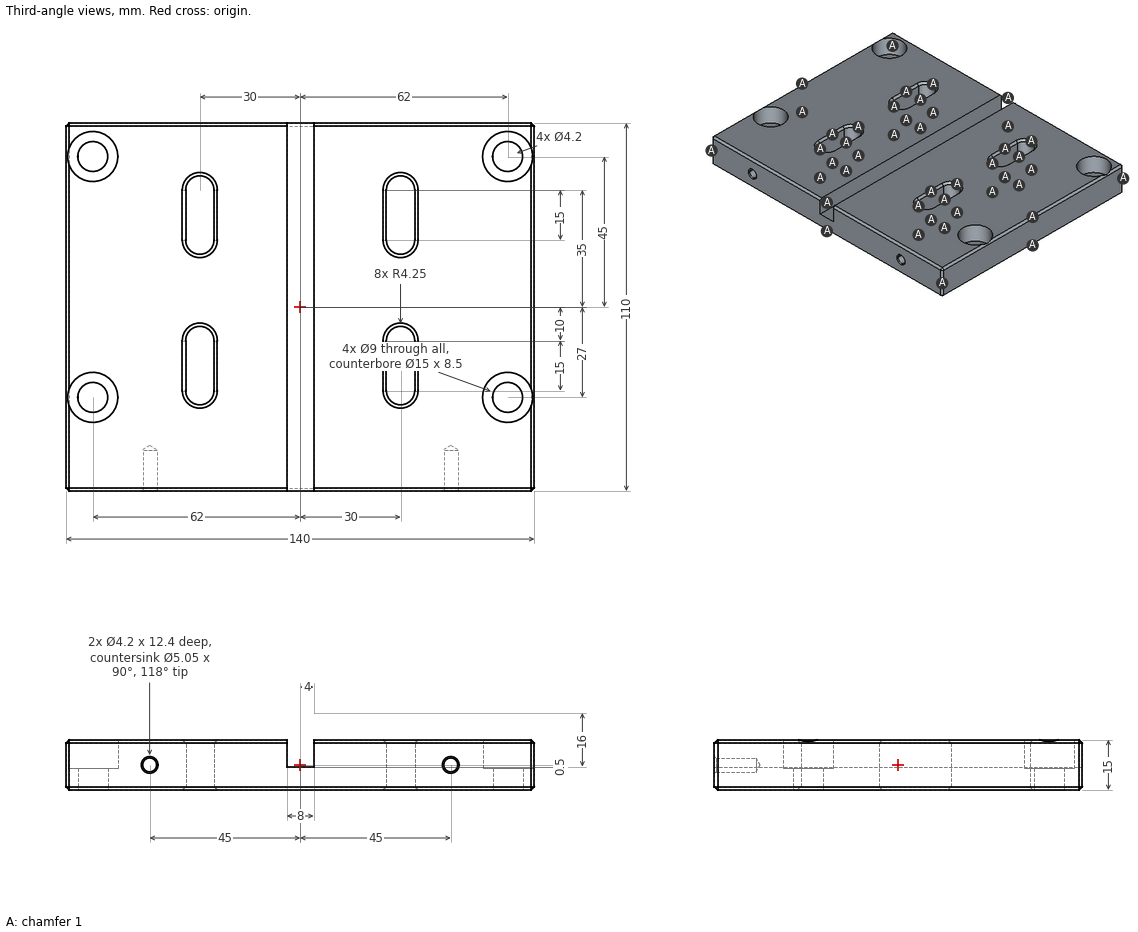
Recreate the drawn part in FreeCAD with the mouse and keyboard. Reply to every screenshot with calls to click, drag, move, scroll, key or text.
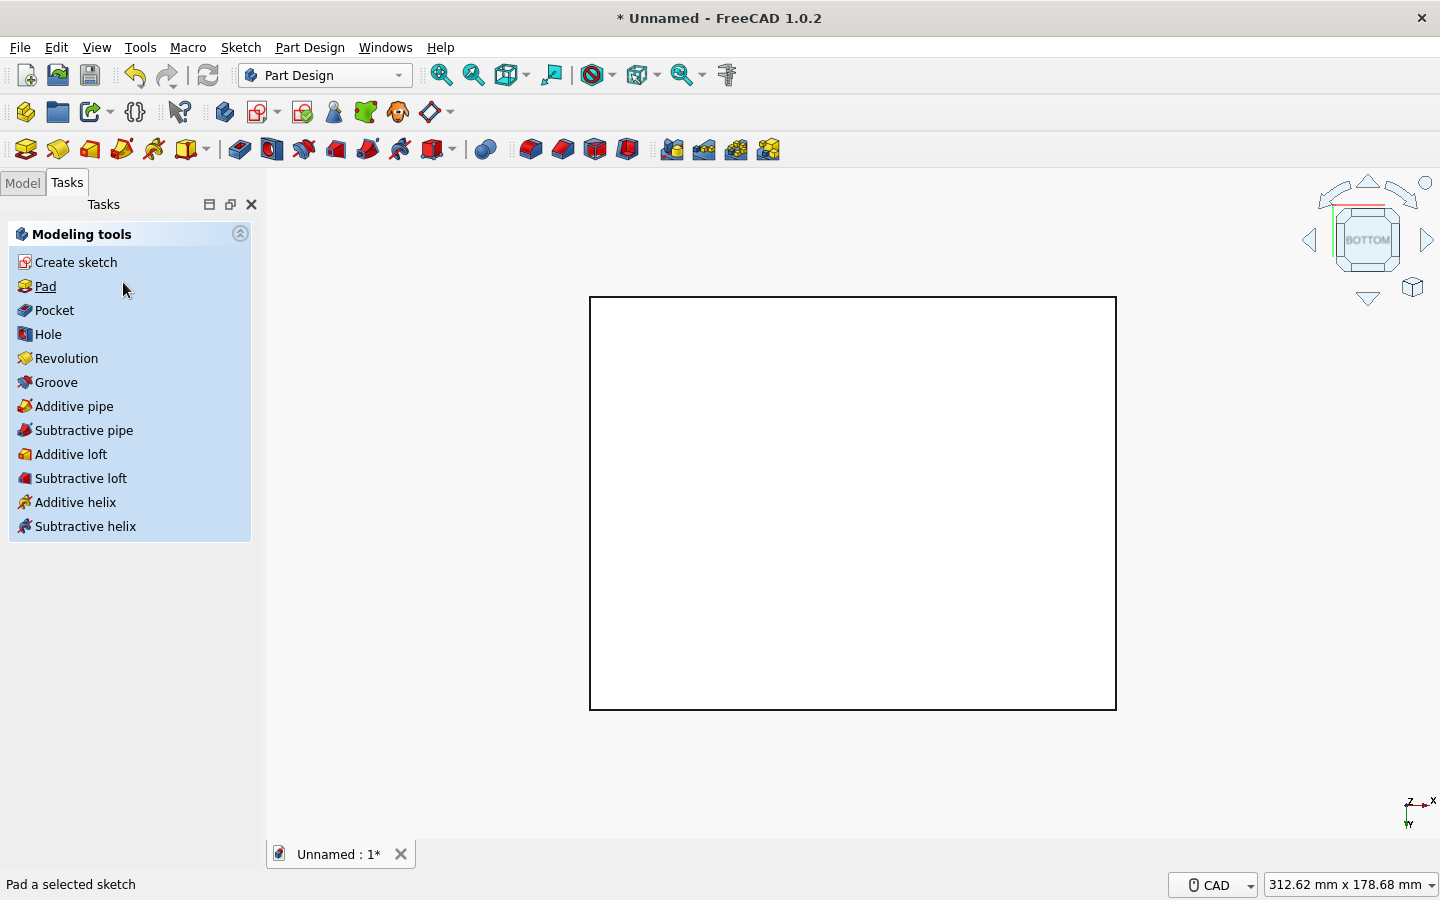
click(240, 150)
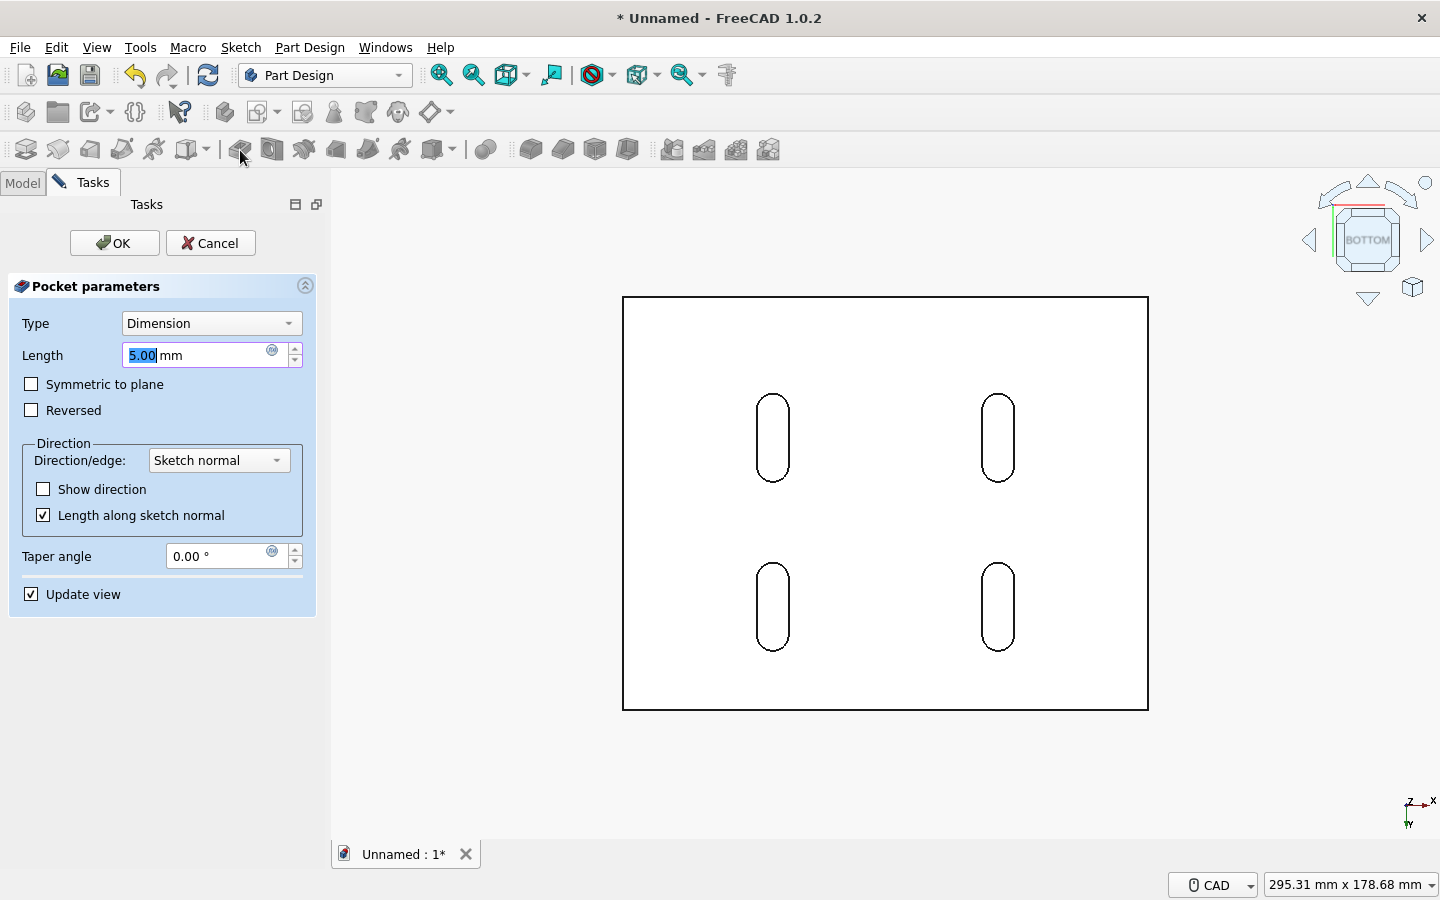
click(212, 324)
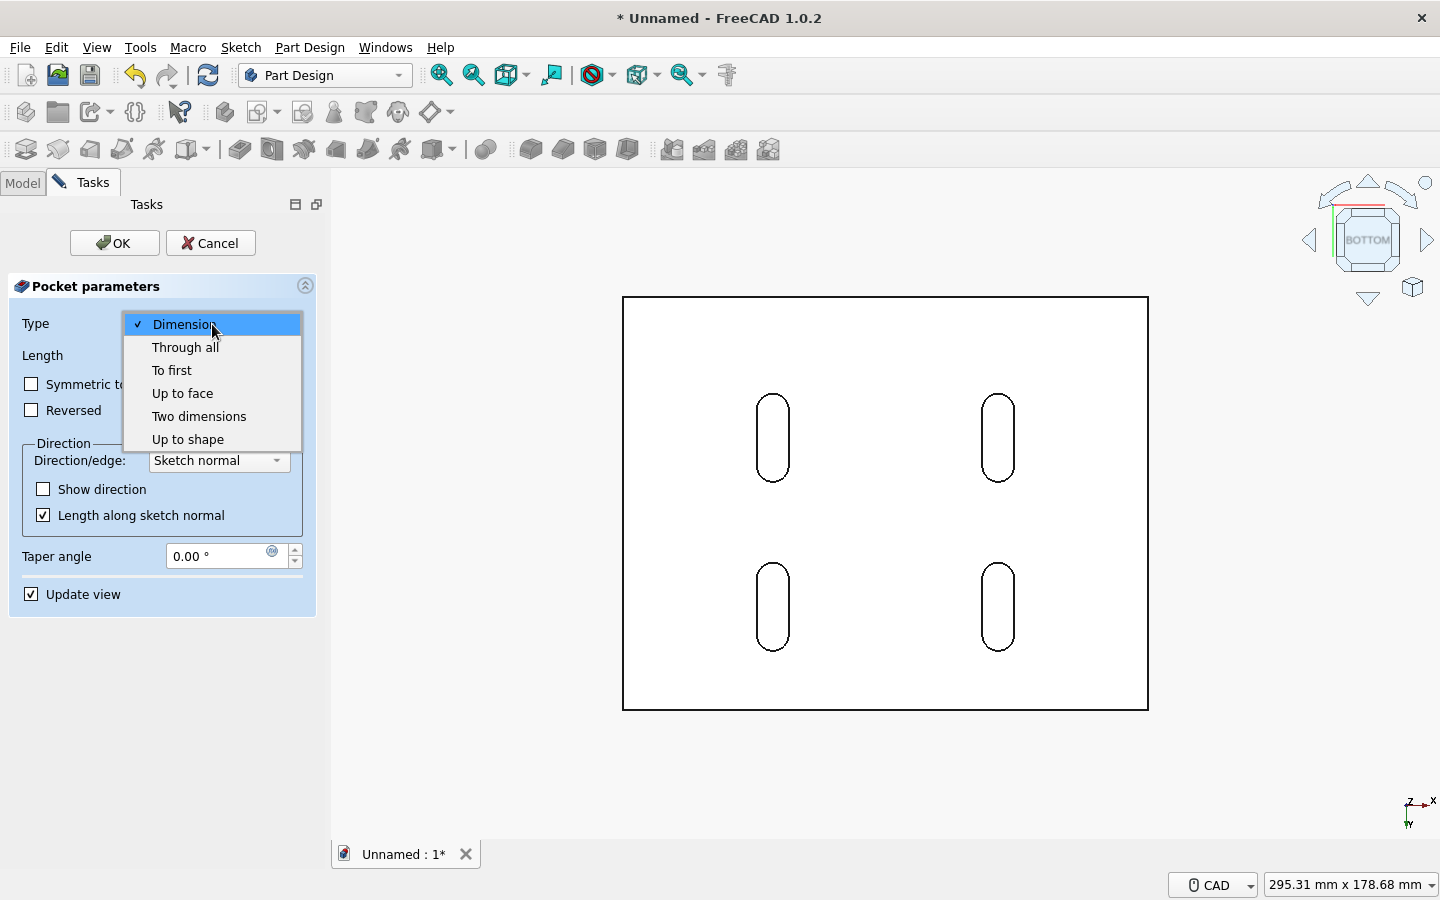
click(212, 348)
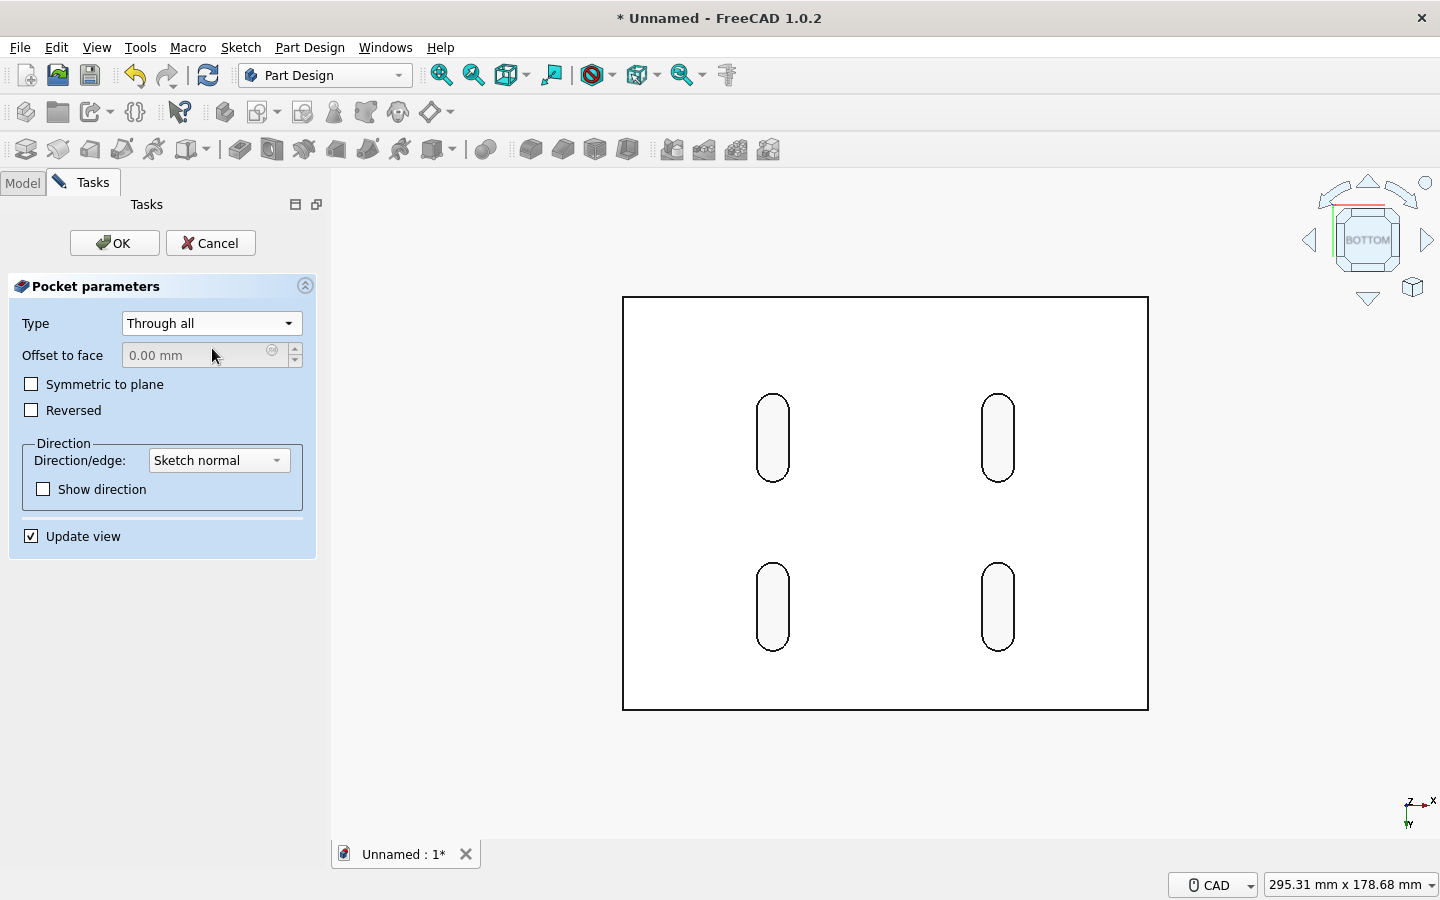
click(115, 243)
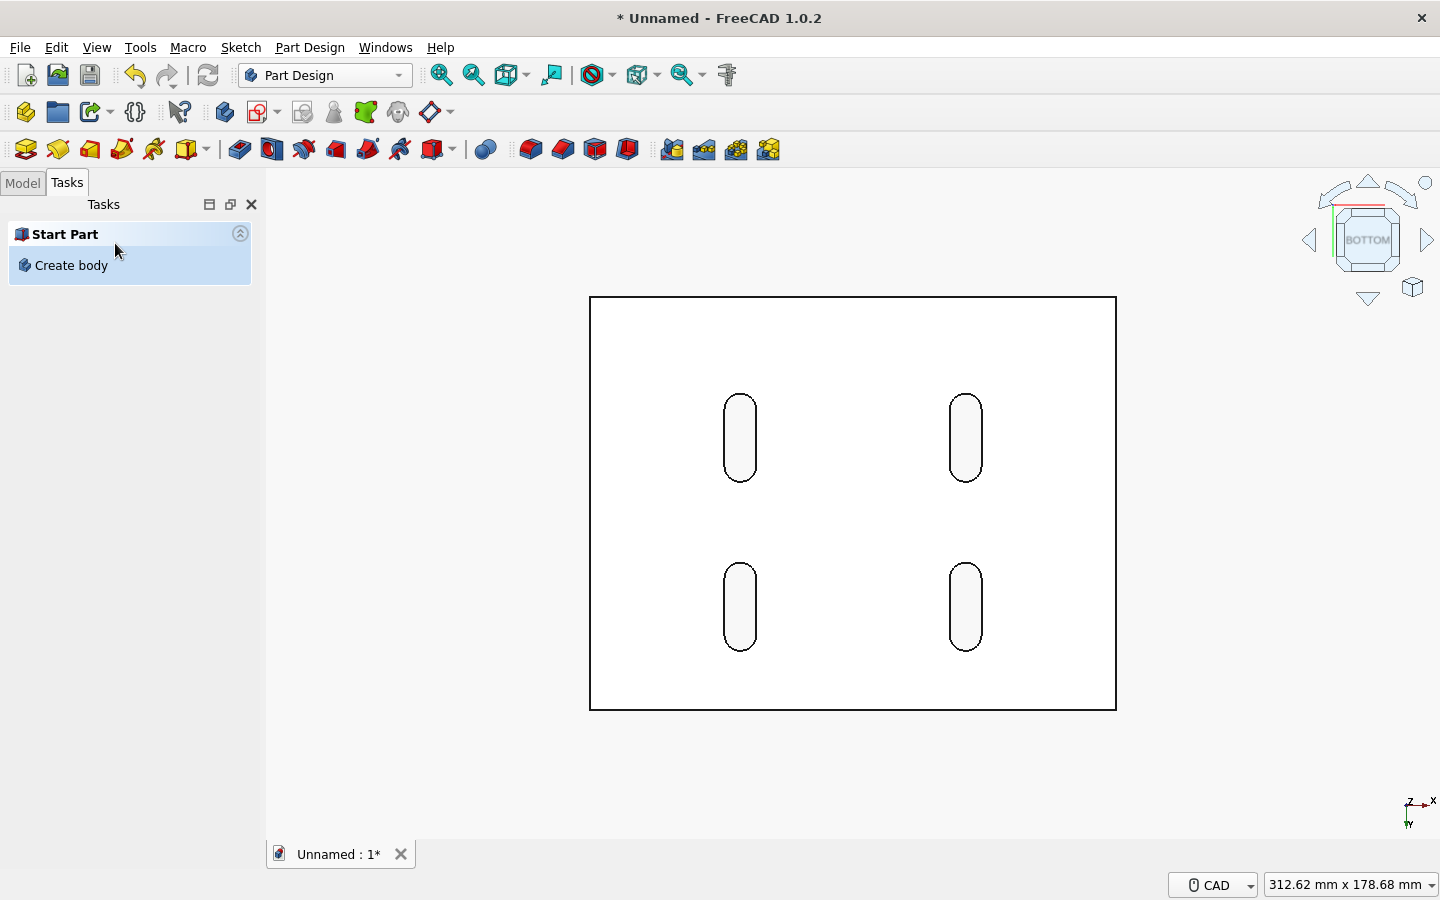
click(853, 503)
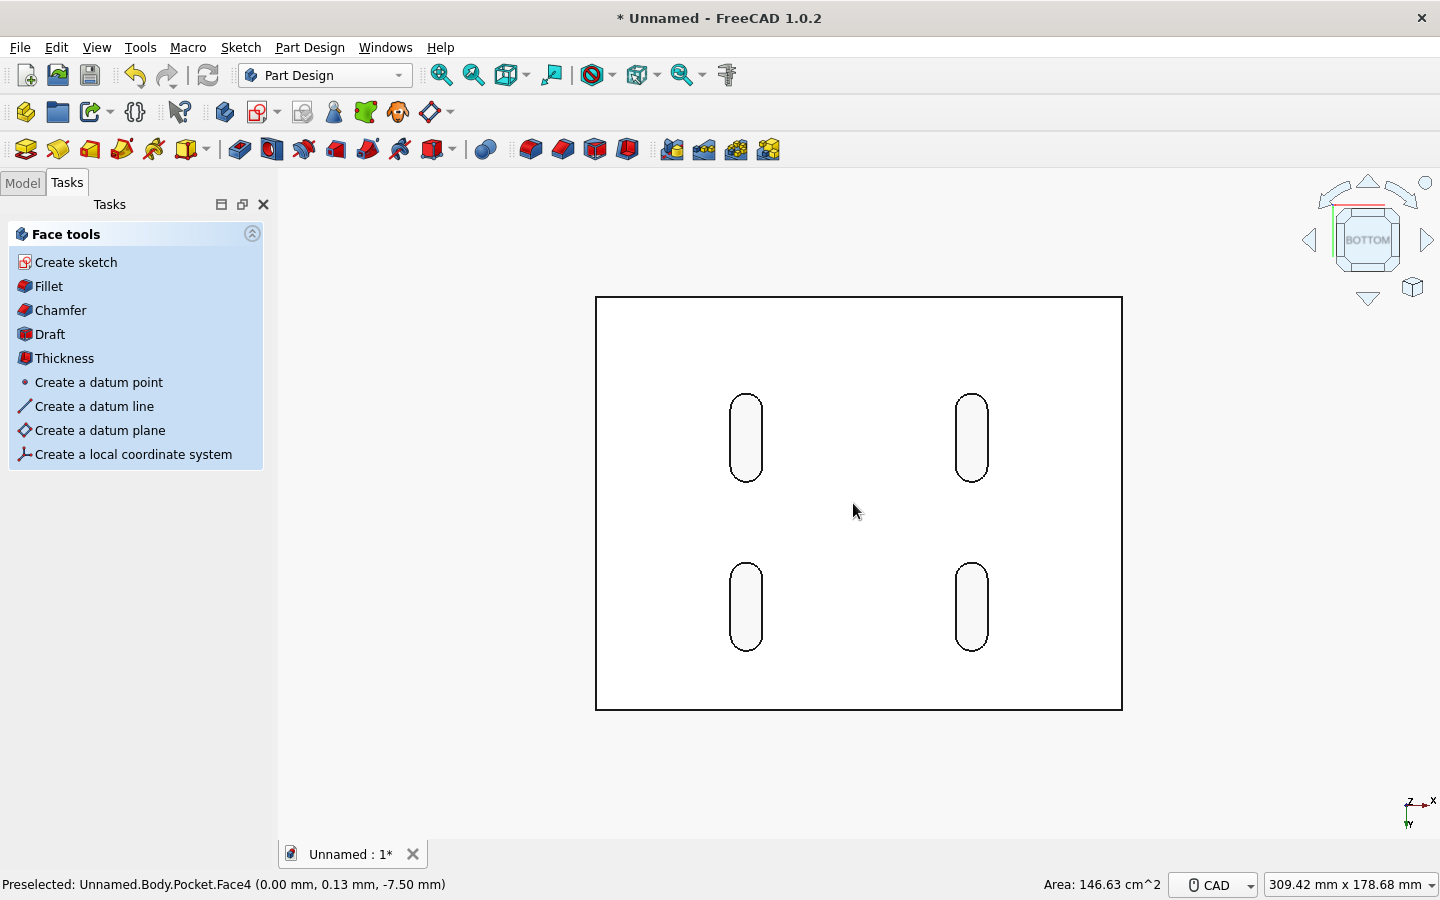
key(0)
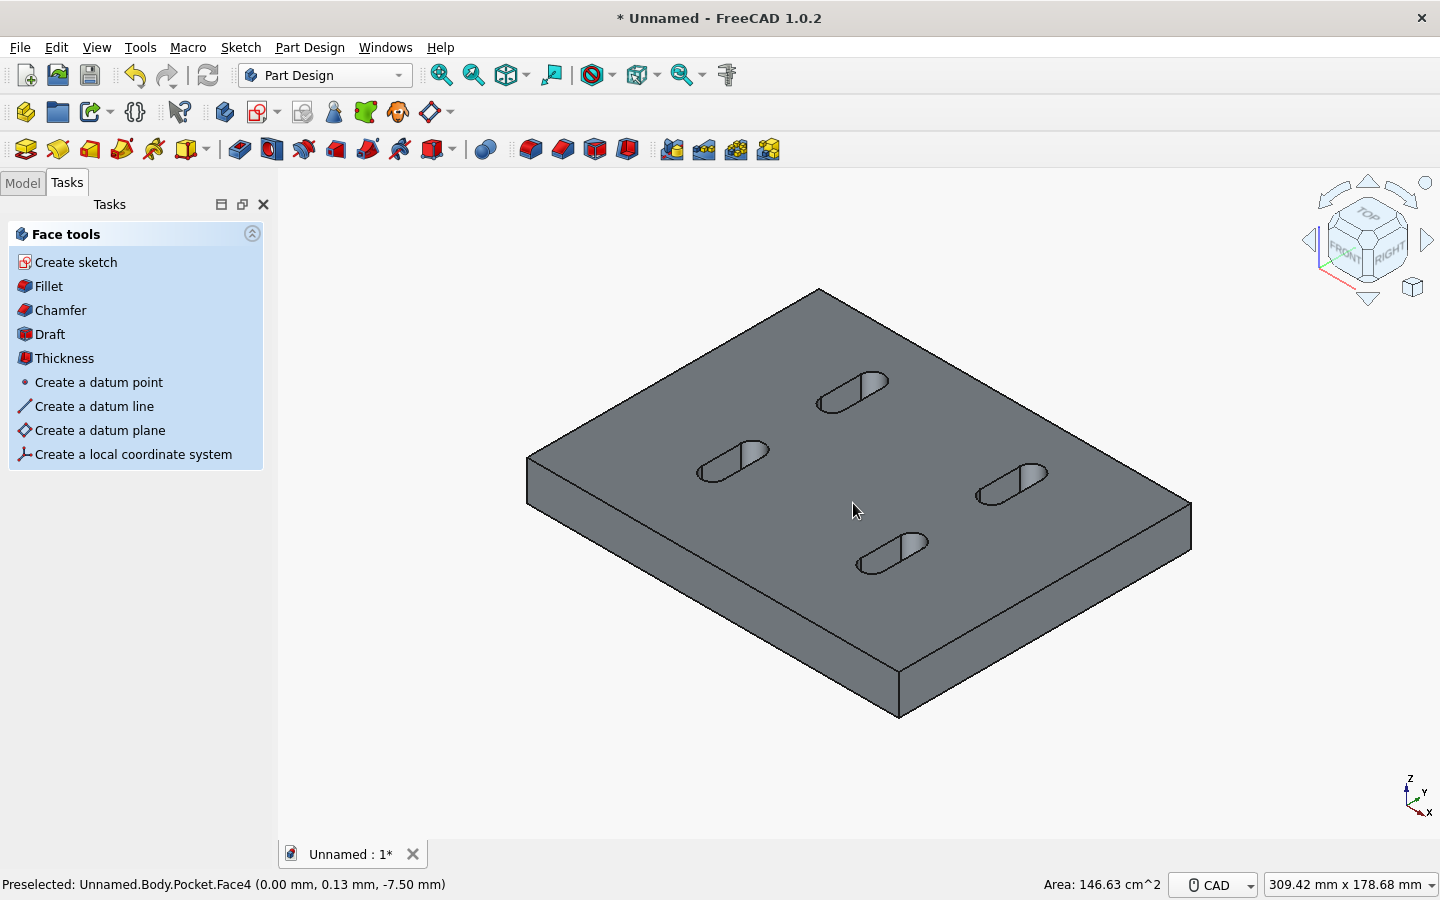
click(859, 480, ctrl)